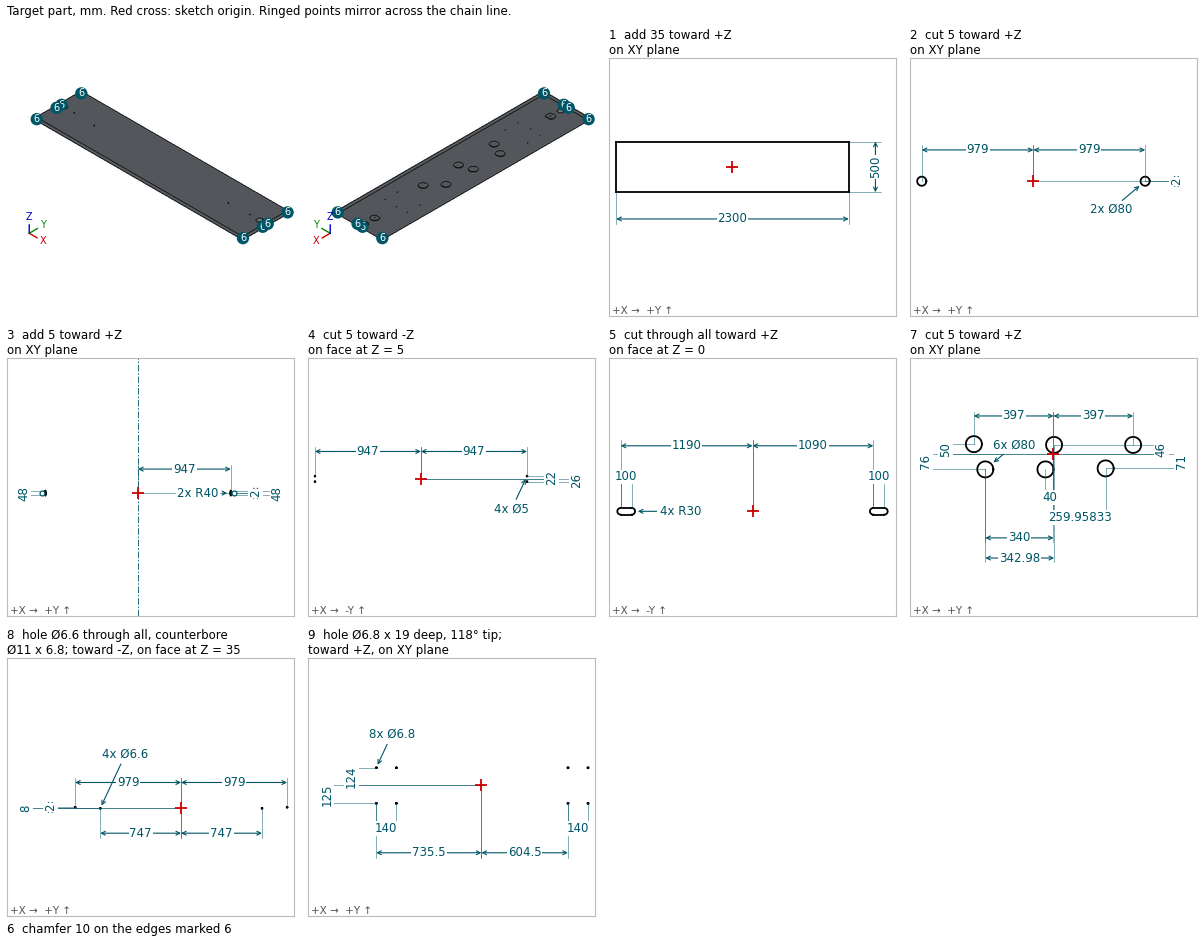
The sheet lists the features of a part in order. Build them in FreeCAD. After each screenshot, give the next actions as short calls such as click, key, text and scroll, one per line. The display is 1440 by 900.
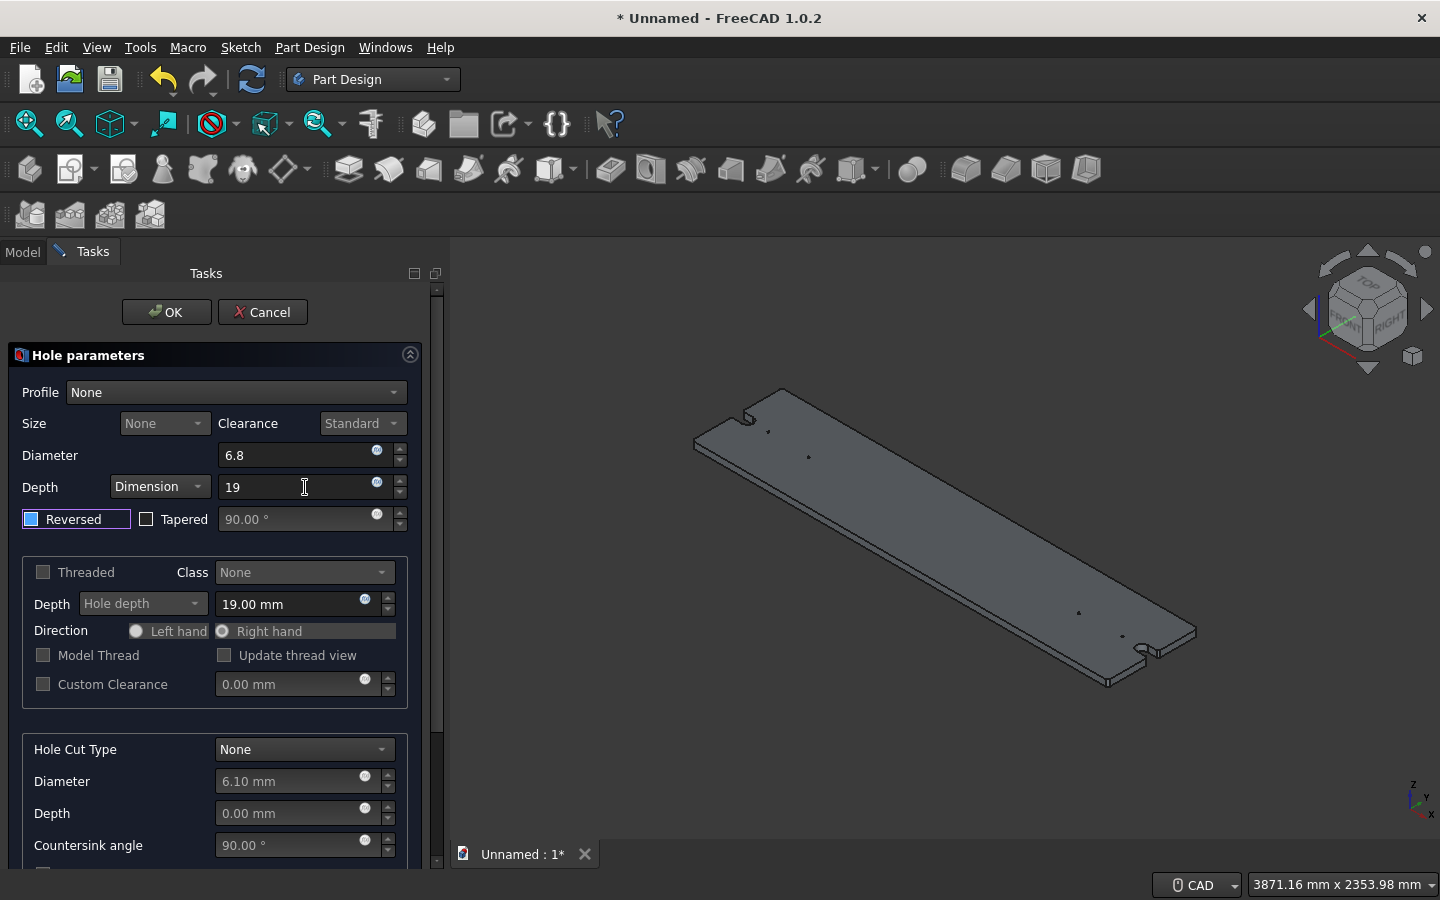
click(30, 519)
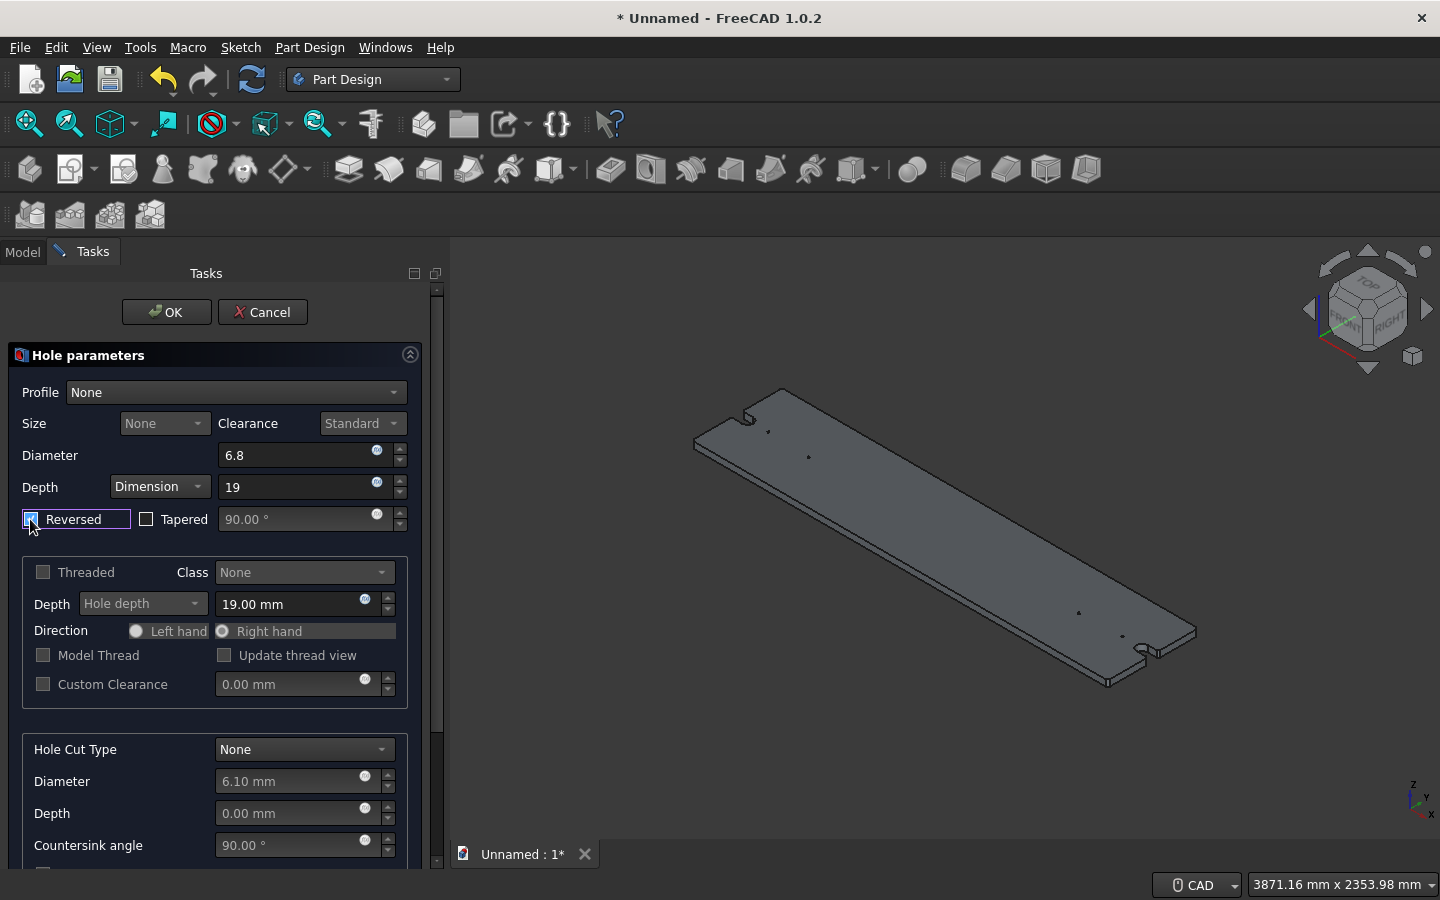
click(167, 312)